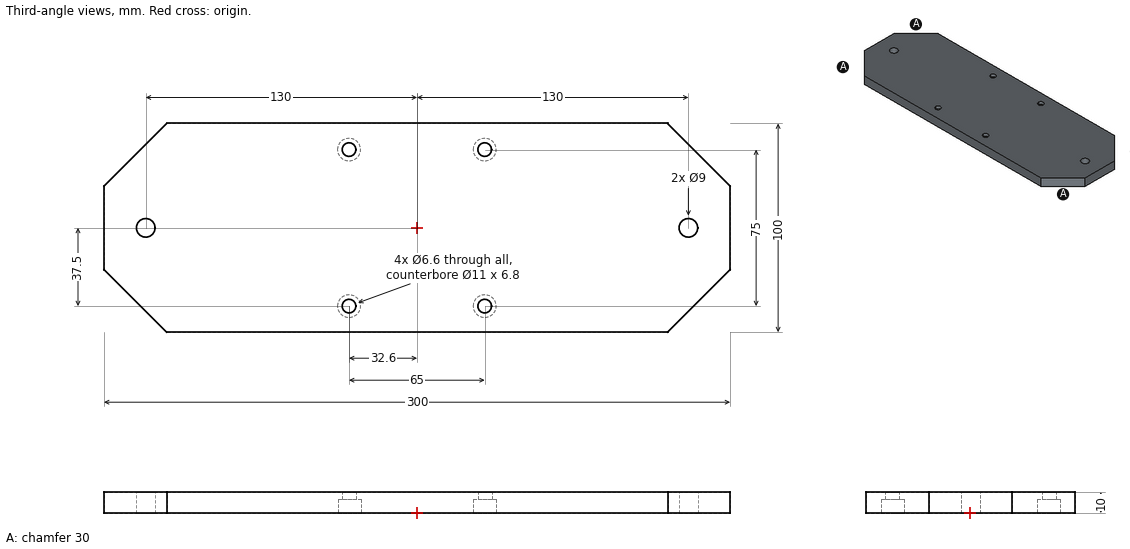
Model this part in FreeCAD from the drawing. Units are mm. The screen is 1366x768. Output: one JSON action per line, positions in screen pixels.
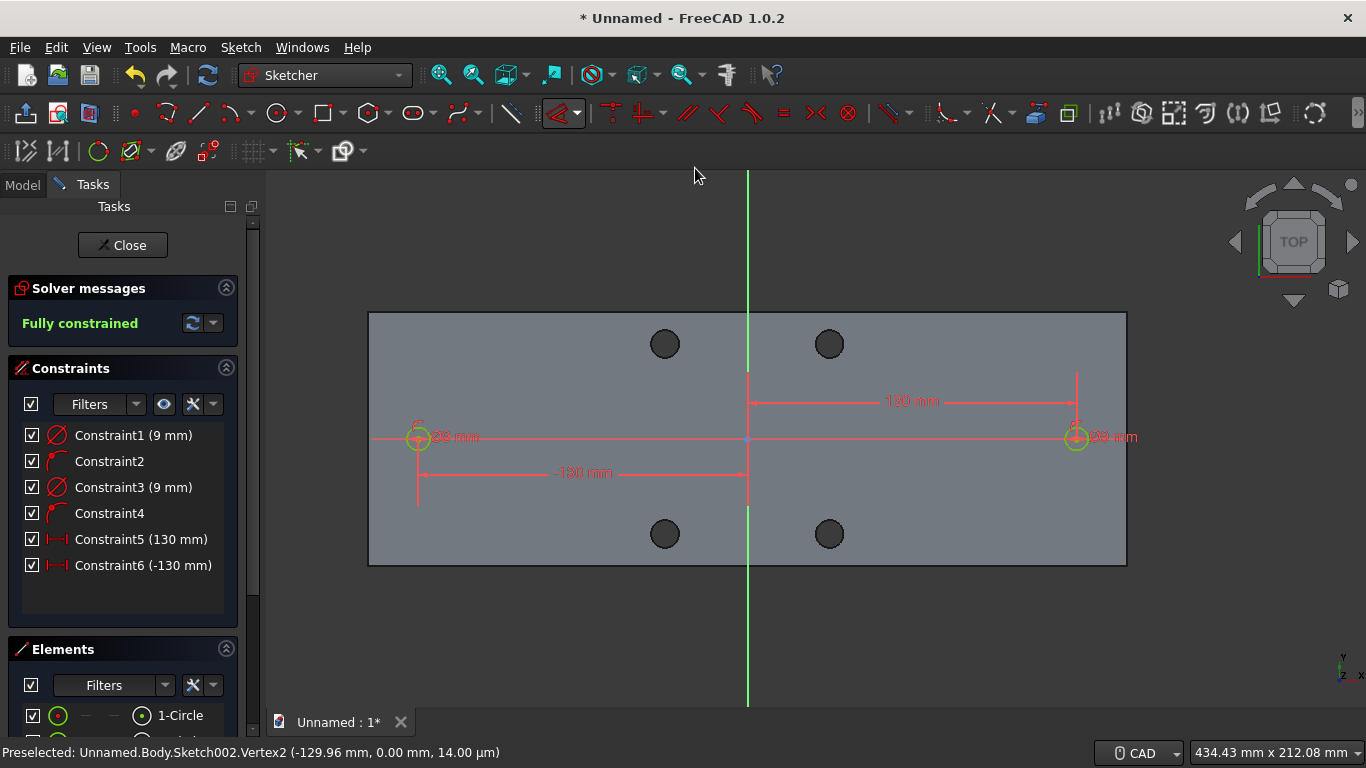
{"action": "left_click", "coordinate": [123, 245]}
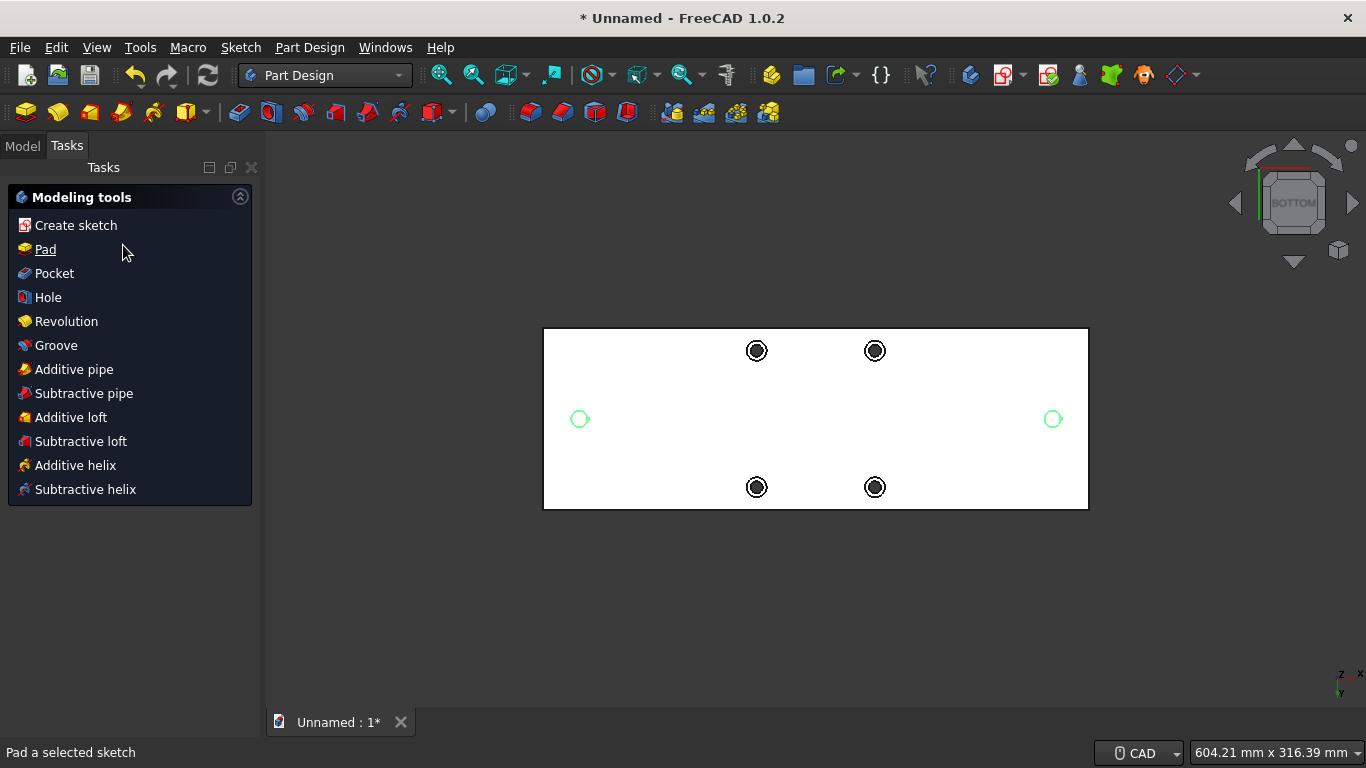
{"action": "left_click", "coordinate": [240, 112]}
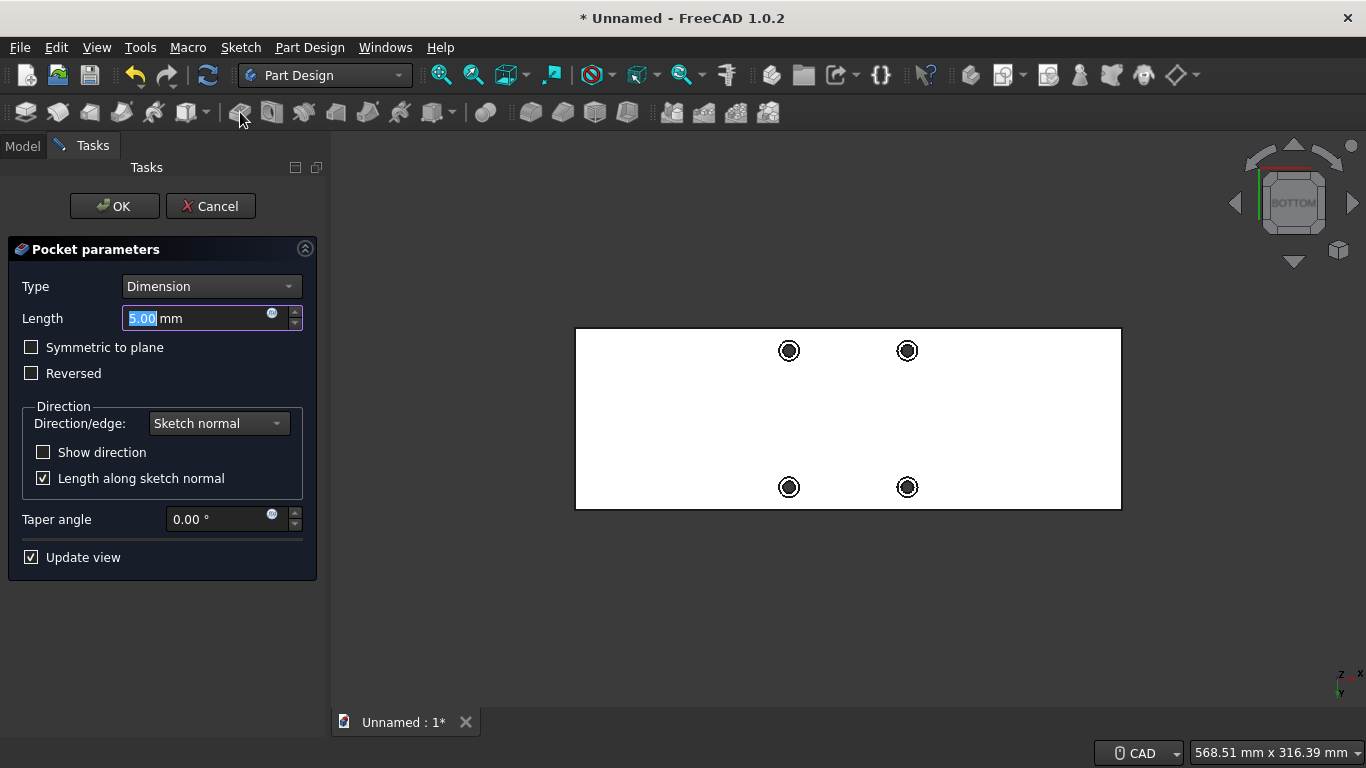
{"action": "left_click", "coordinate": [212, 286]}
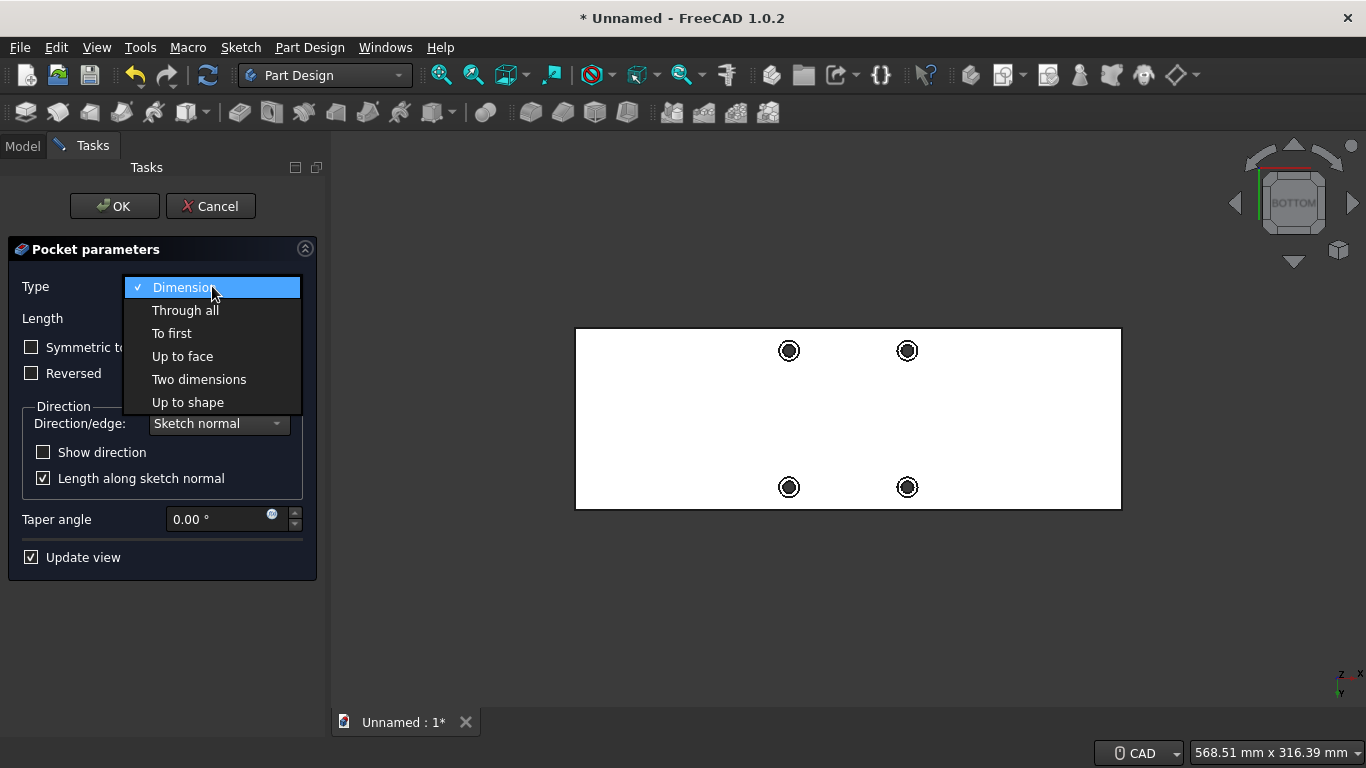
{"action": "left_click", "coordinate": [212, 310]}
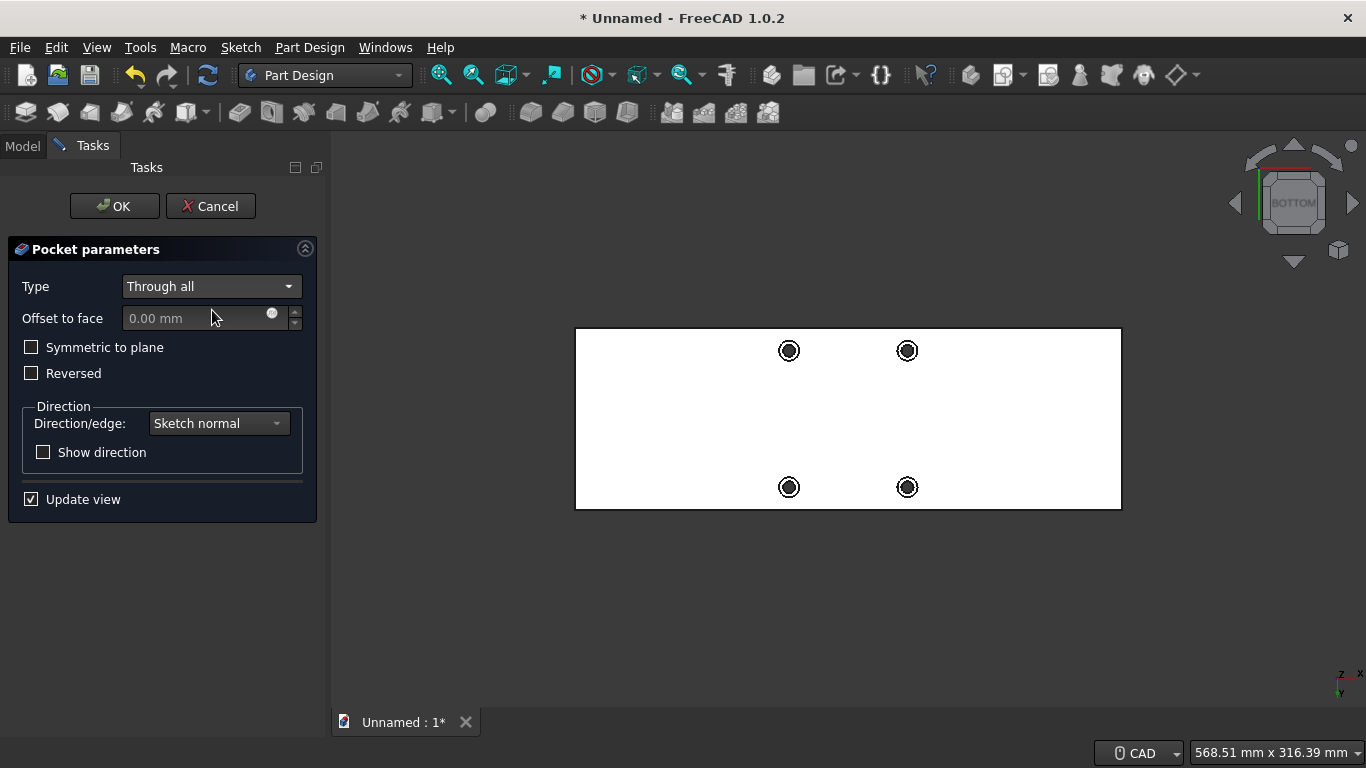
{"action": "left_click", "coordinate": [30, 373]}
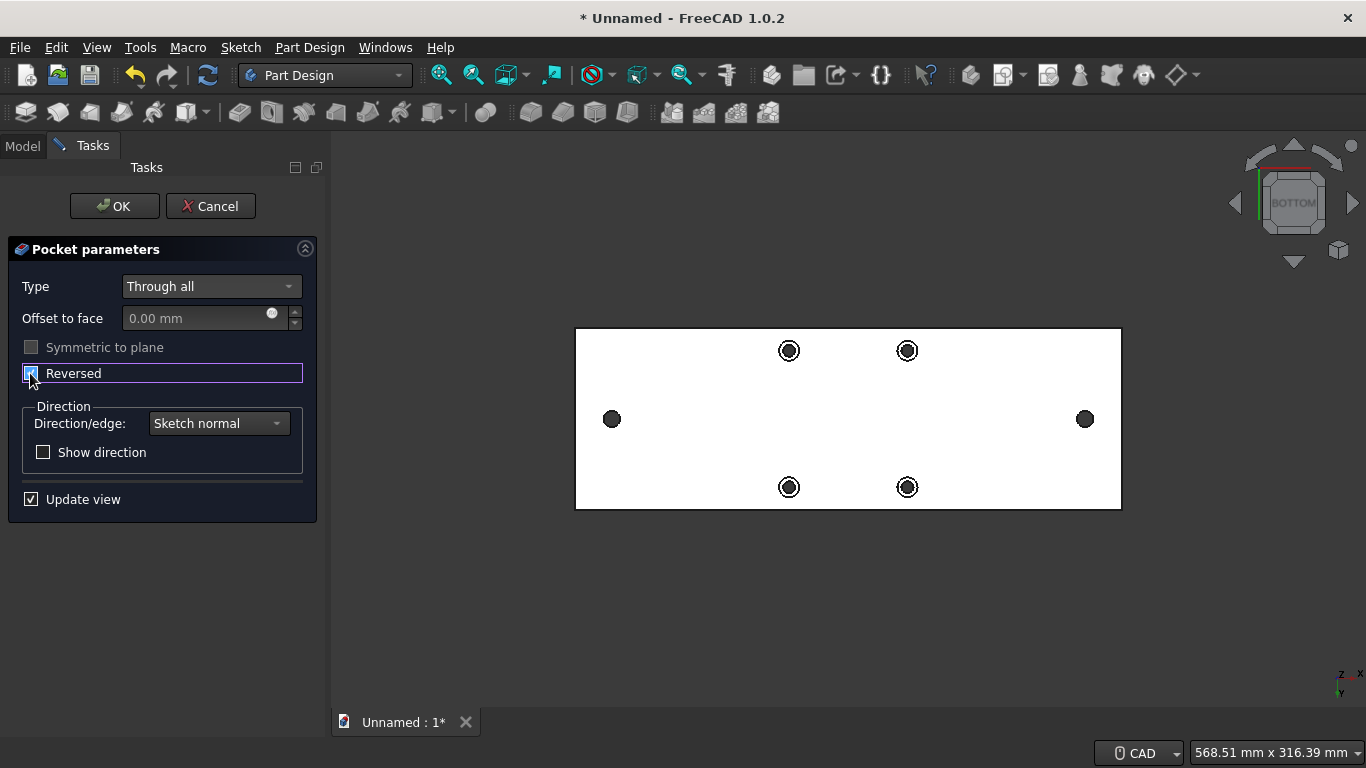
{"action": "left_click", "coordinate": [115, 206]}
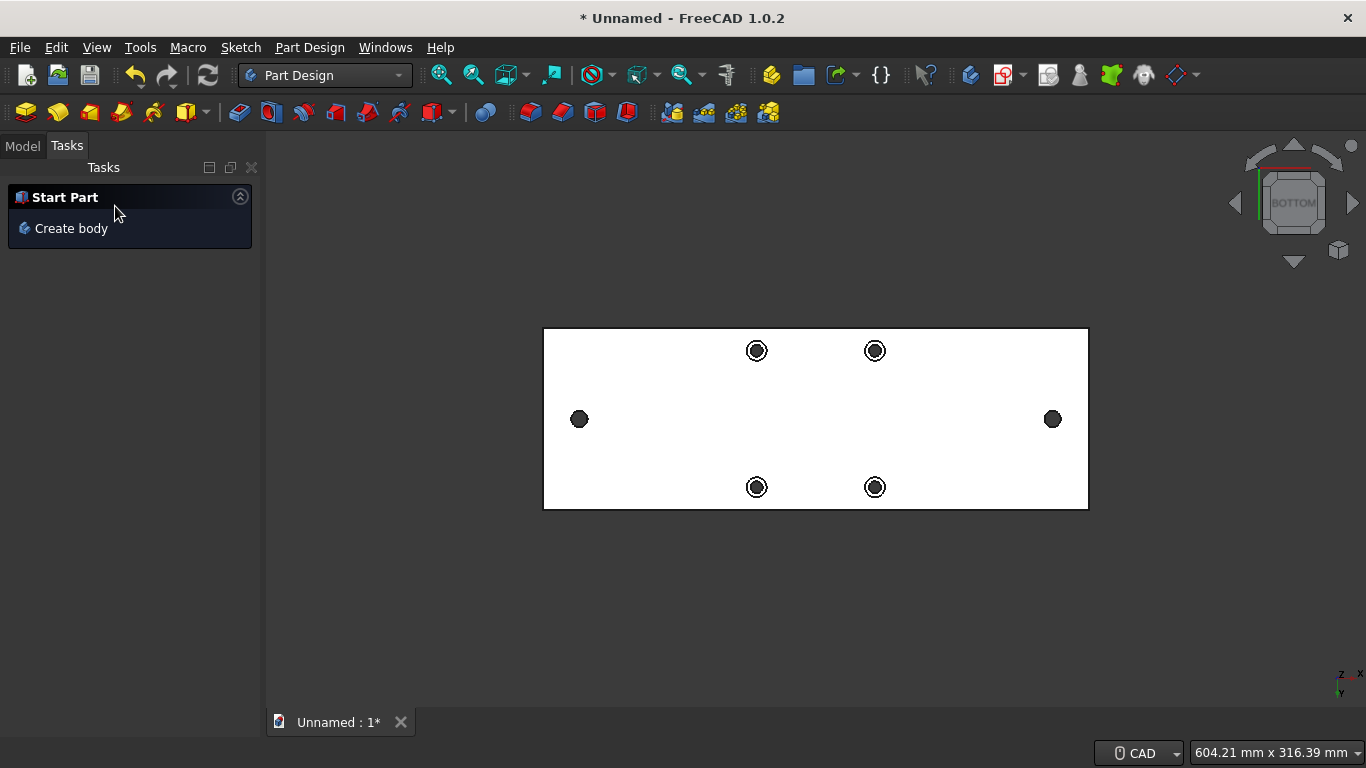
{"action": "scroll", "coordinate": [543, 509], "scroll_direction": "up", "scroll_amount": 4}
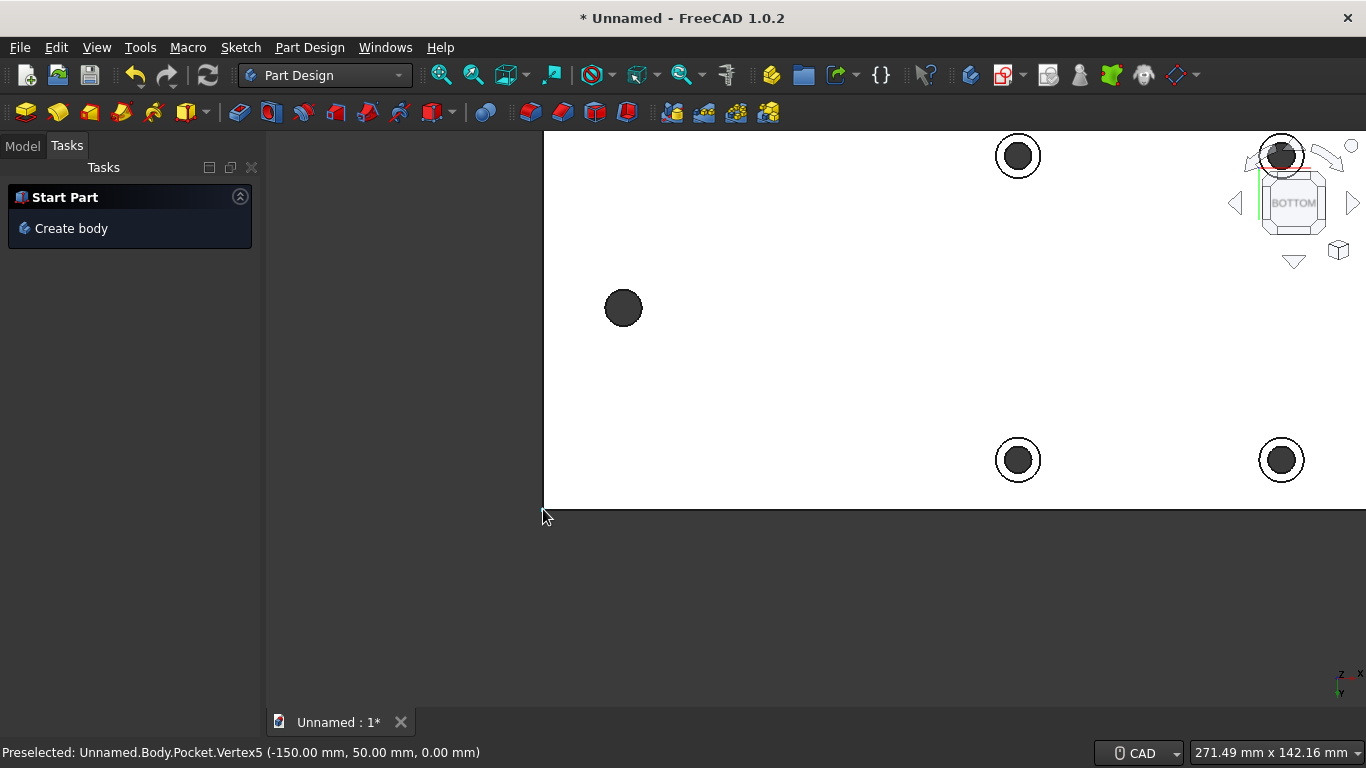
{"action": "key", "text": "v f"}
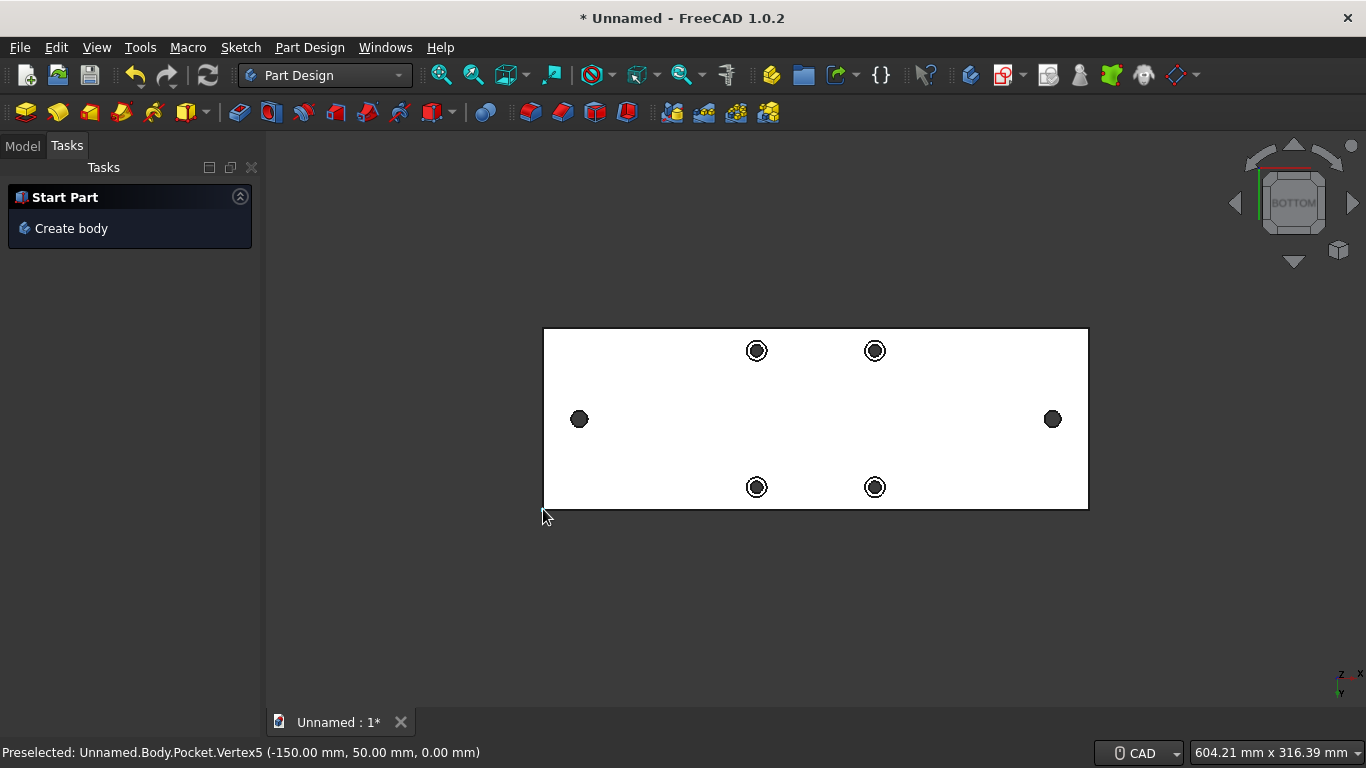
{"action": "key", "text": "0"}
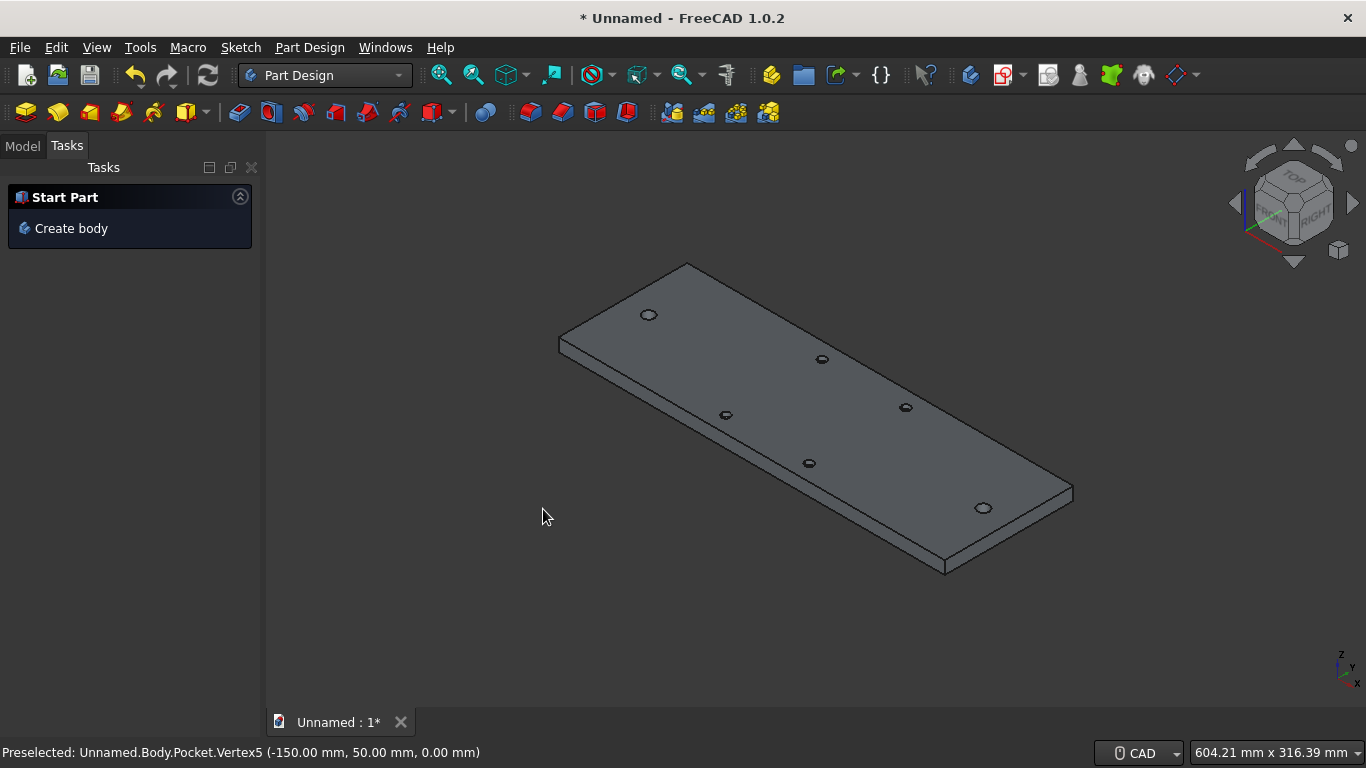
{"action": "left_click", "coordinate": [945, 567]}